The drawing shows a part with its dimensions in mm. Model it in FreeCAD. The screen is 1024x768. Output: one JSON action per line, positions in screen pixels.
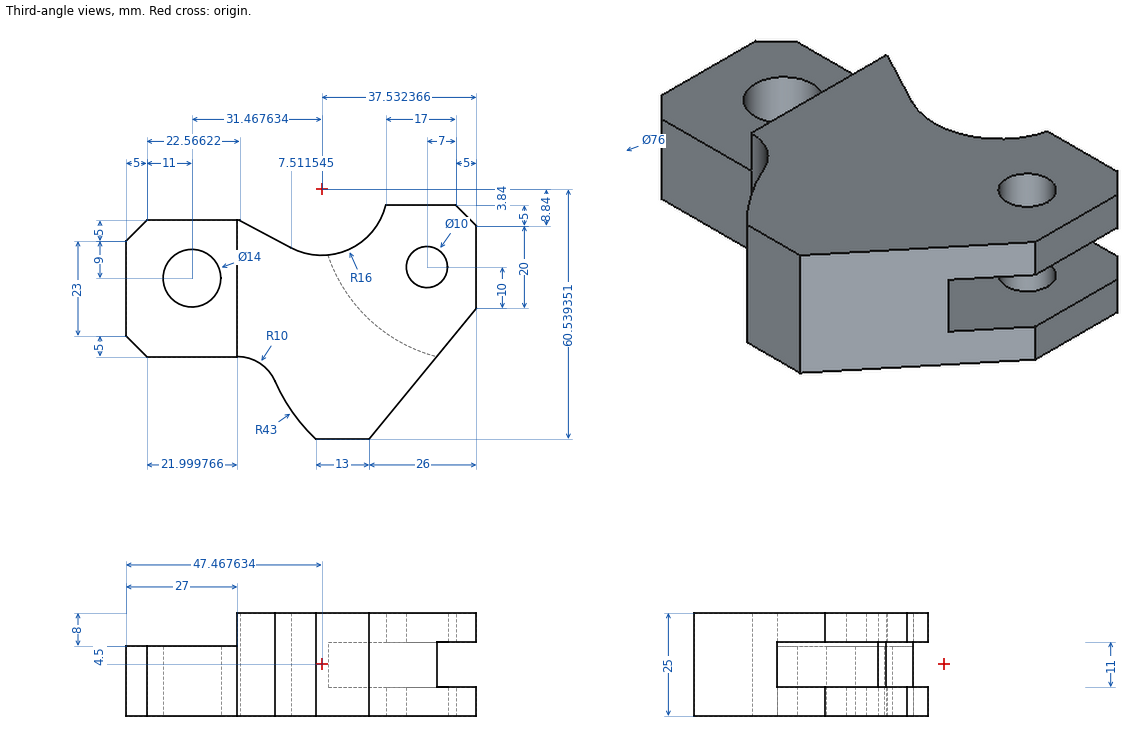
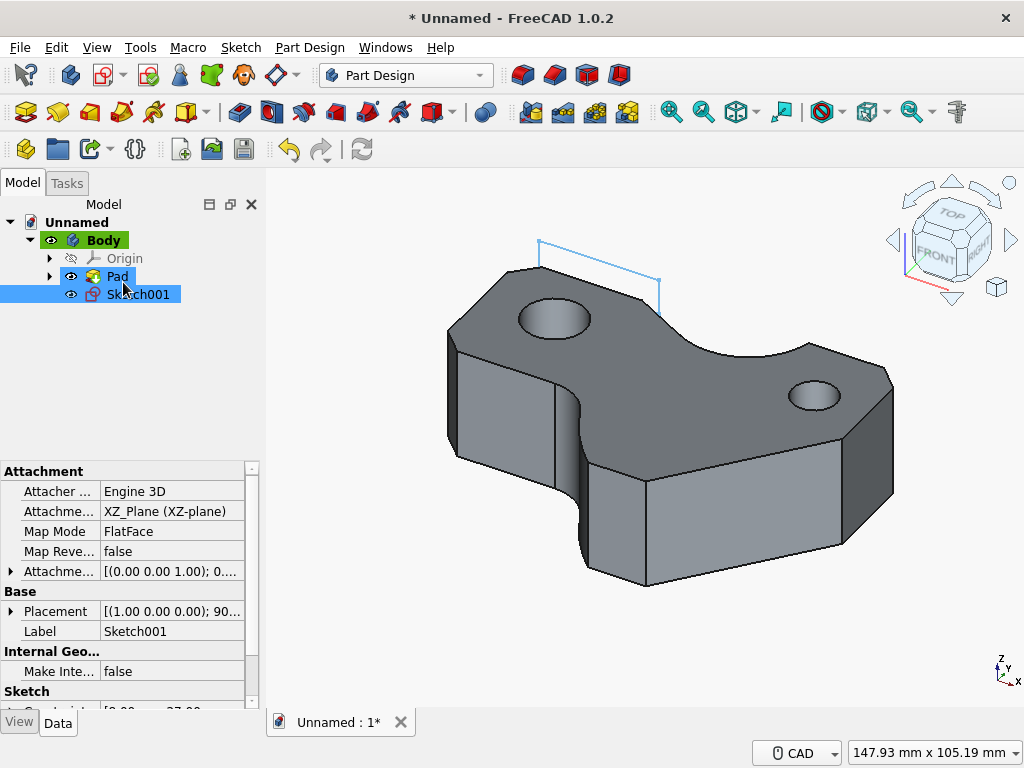
{"action": "left_click", "coordinate": [240, 112]}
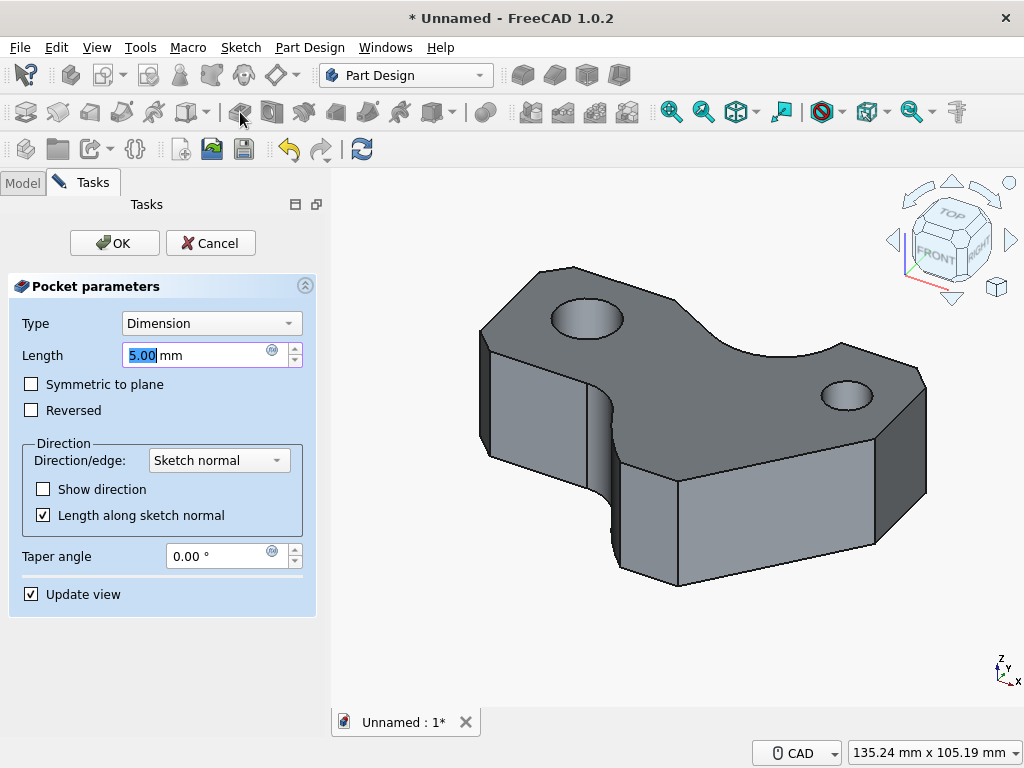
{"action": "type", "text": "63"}
{"action": "key", "text": "Tab"}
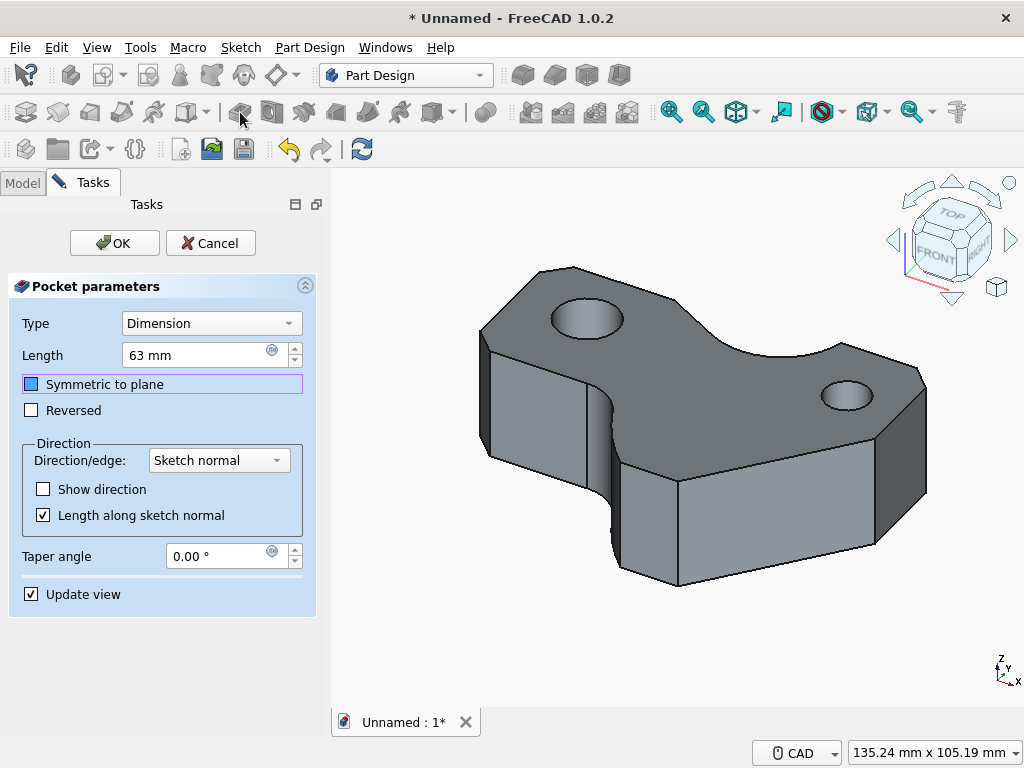
{"action": "left_click", "coordinate": [30, 410]}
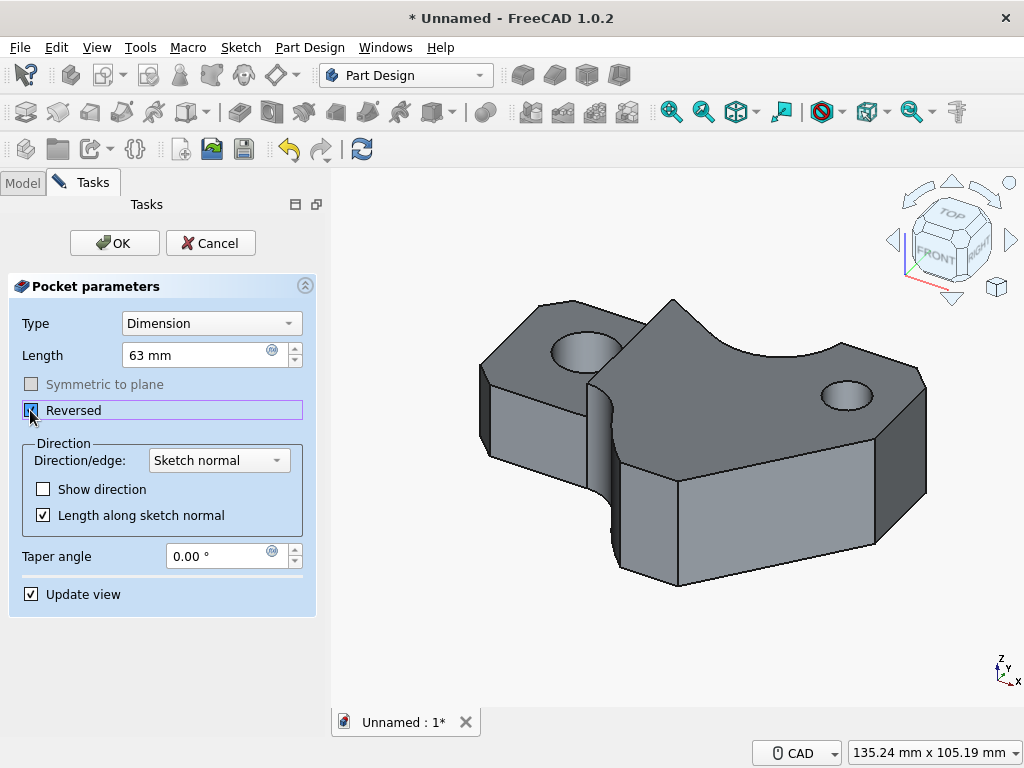
{"action": "left_click", "coordinate": [115, 243]}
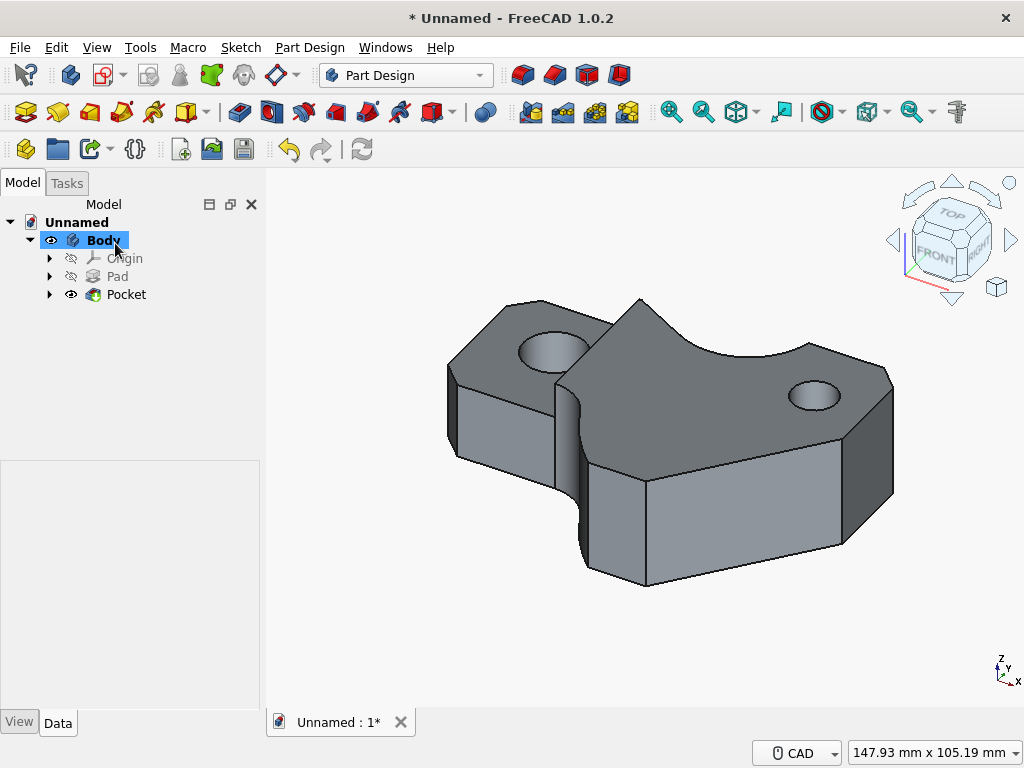
{"action": "left_click", "coordinate": [104, 76]}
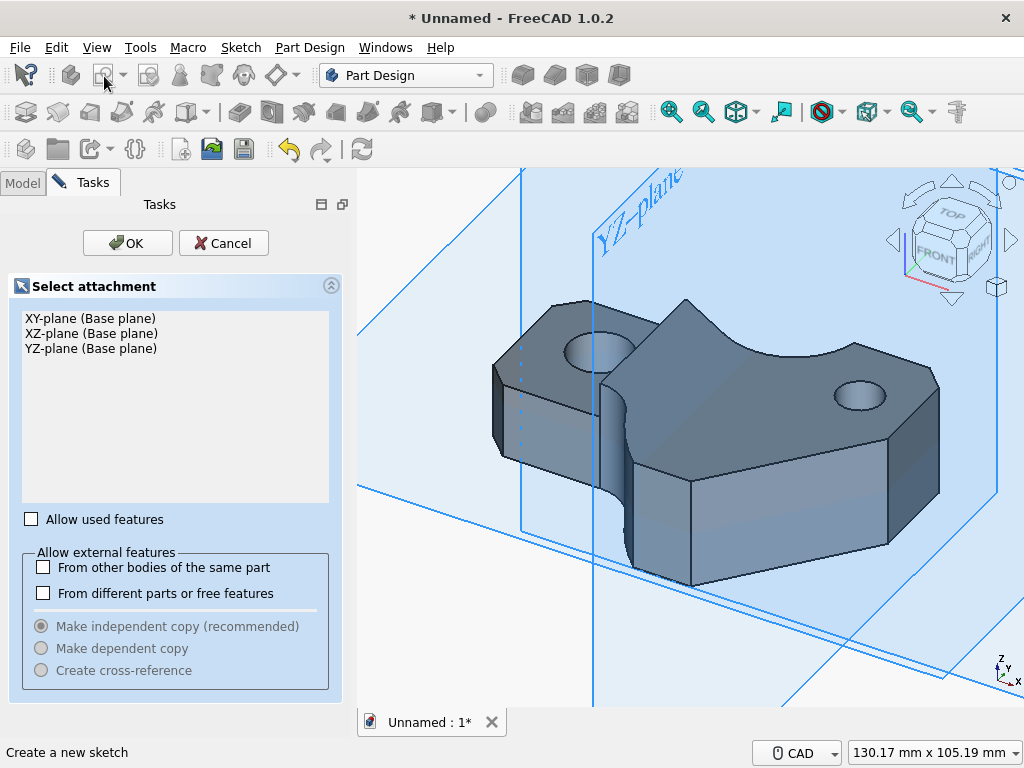
{"action": "left_click", "coordinate": [82, 318]}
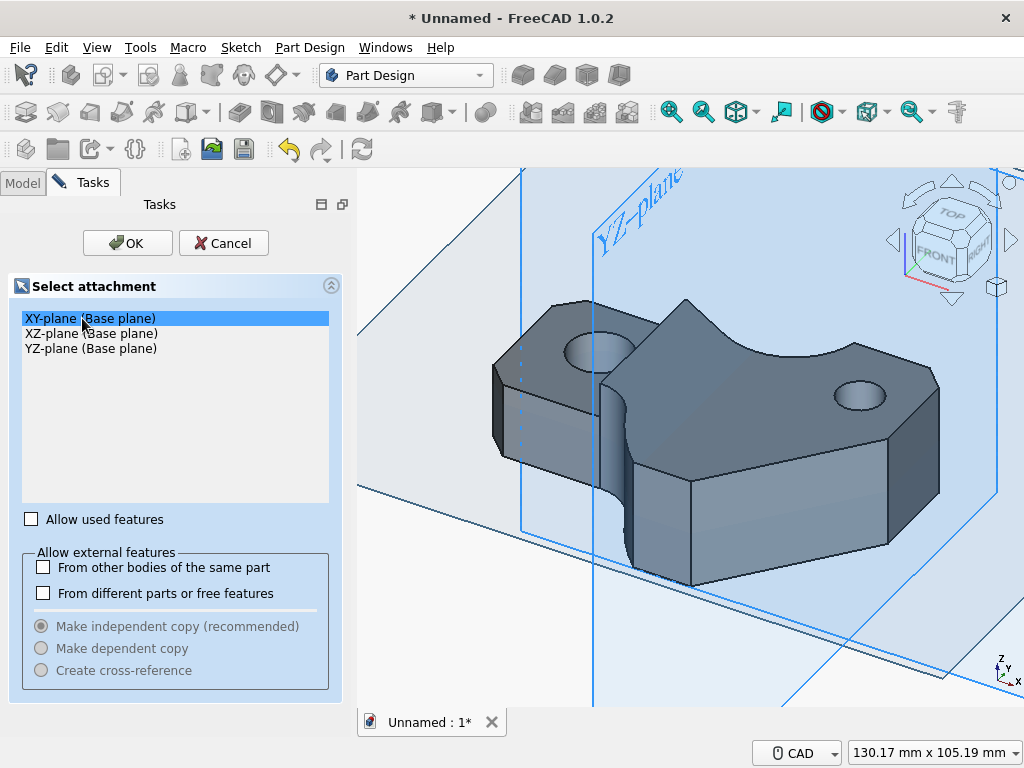
{"action": "left_click", "coordinate": [128, 243]}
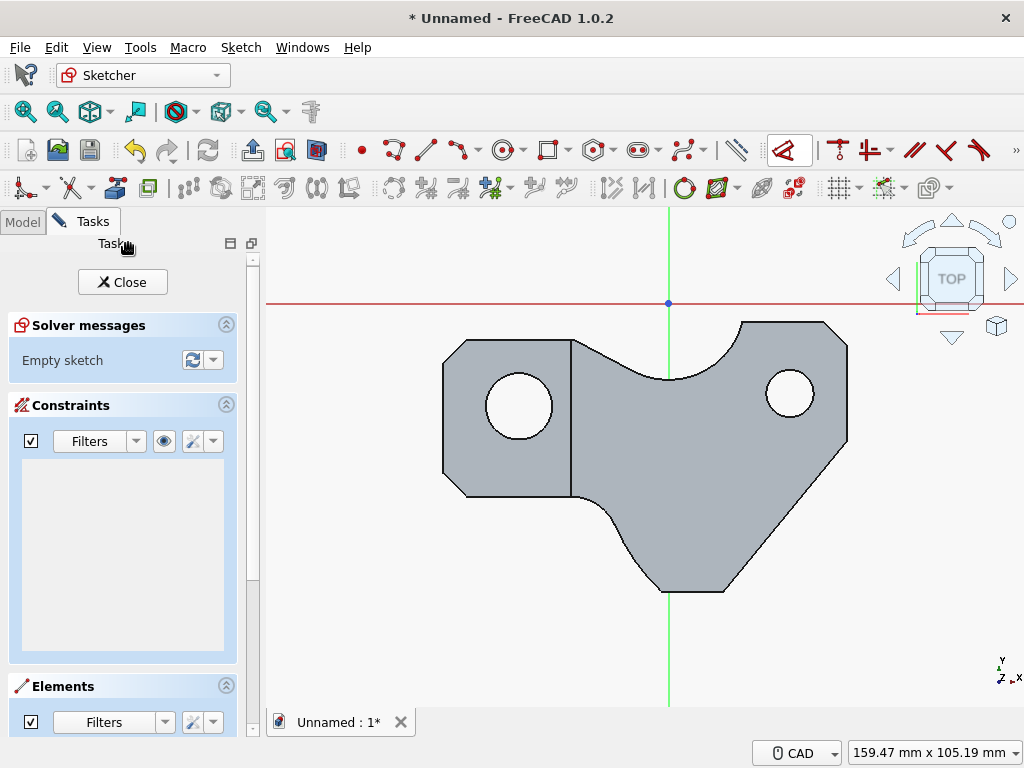
{"action": "left_click", "coordinate": [318, 150]}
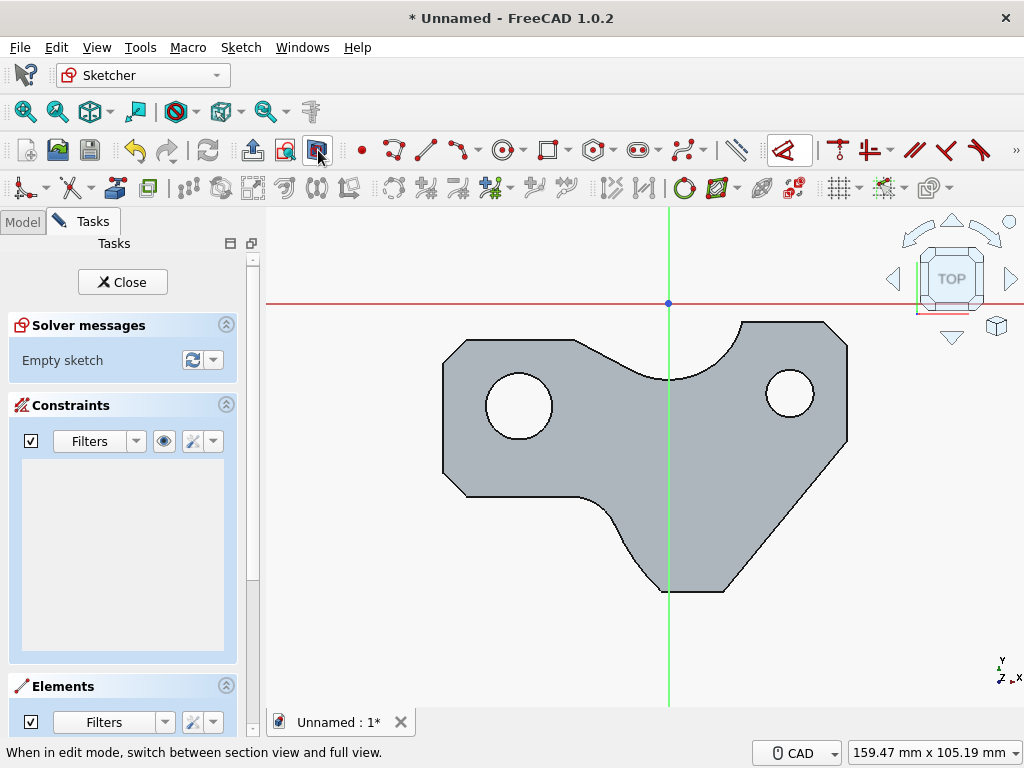
{"action": "scroll", "coordinate": [294, 679], "scroll_direction": "down", "scroll_amount": 2}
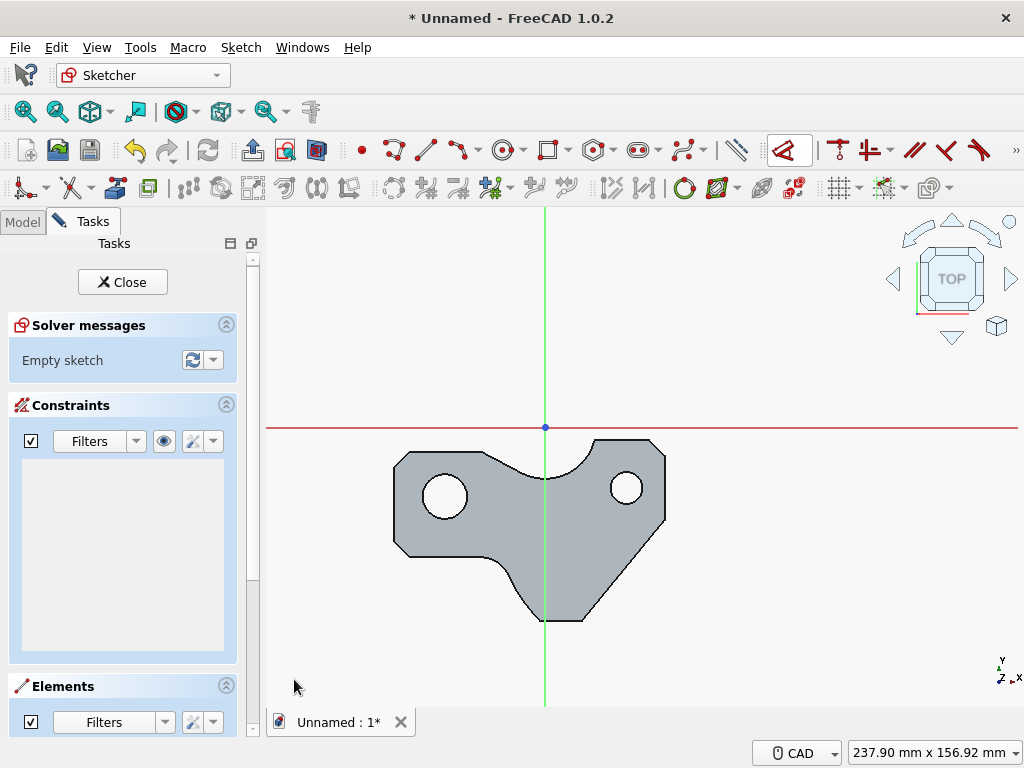
{"action": "left_click", "coordinate": [504, 150]}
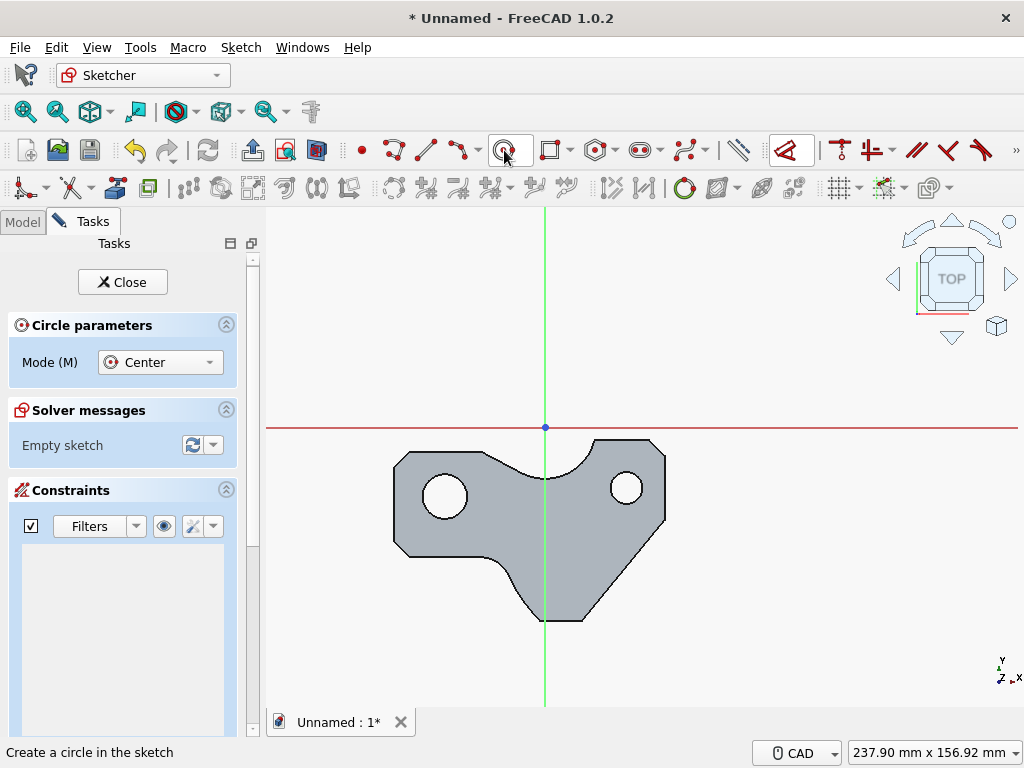
{"action": "scroll", "coordinate": [665, 440], "scroll_direction": "up", "scroll_amount": 2}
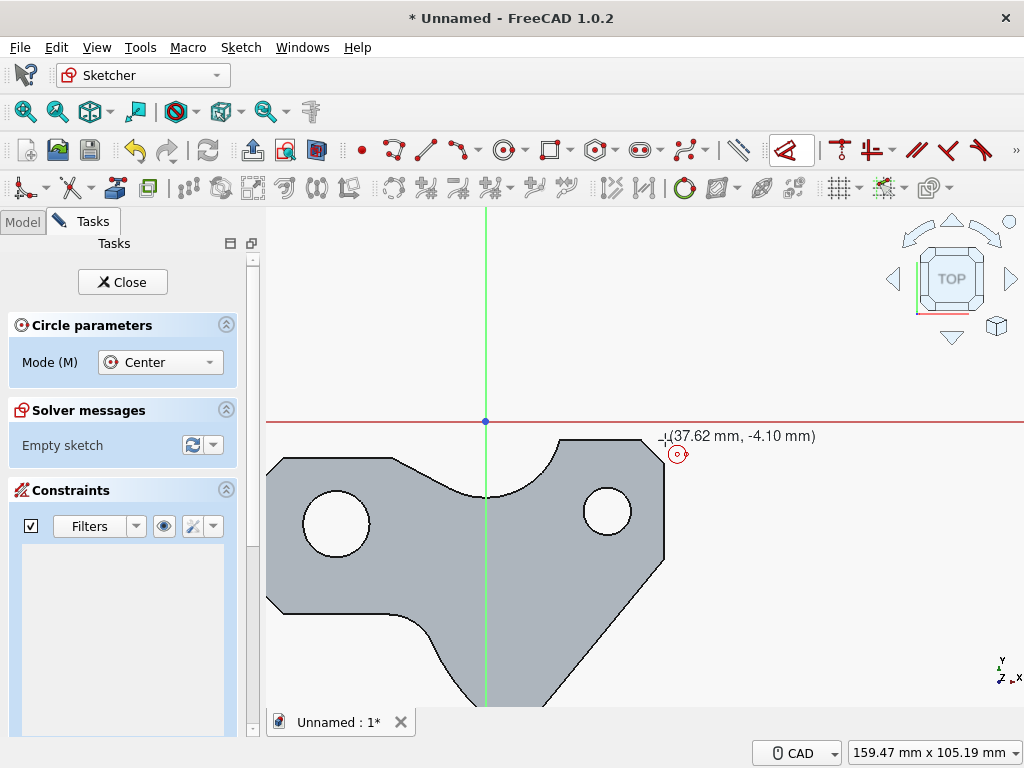
{"action": "left_click", "coordinate": [664, 440]}
{"action": "left_click", "coordinate": [792, 312]}
{"action": "key", "text": "Escape"}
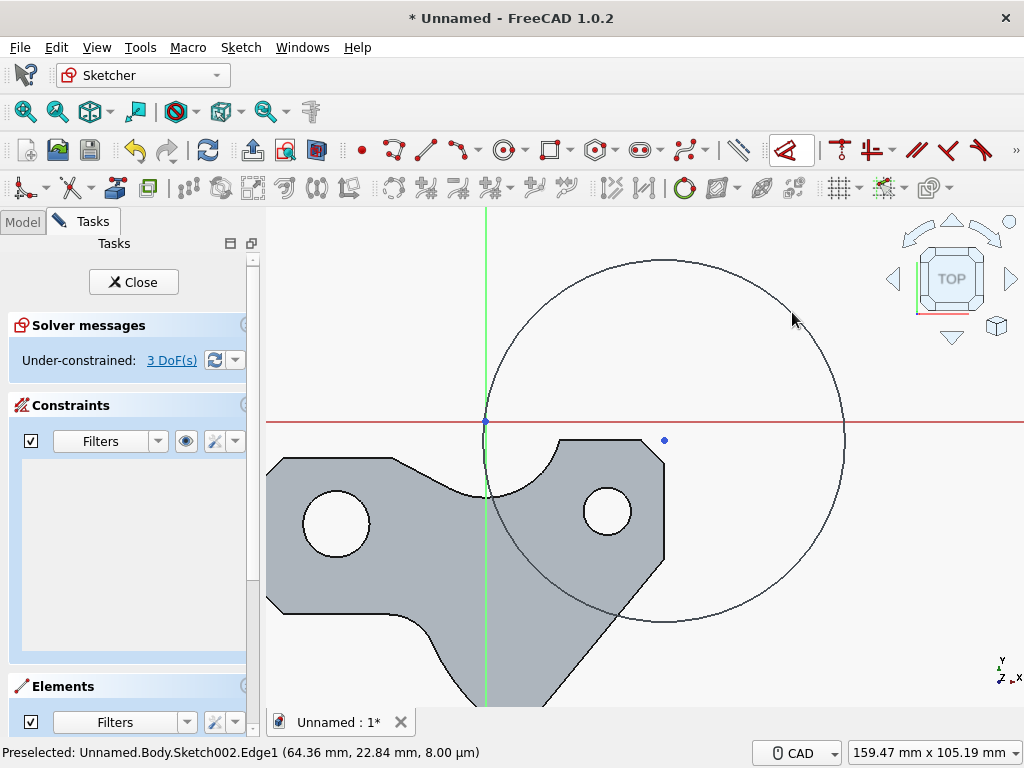
{"action": "left_click", "coordinate": [792, 313]}